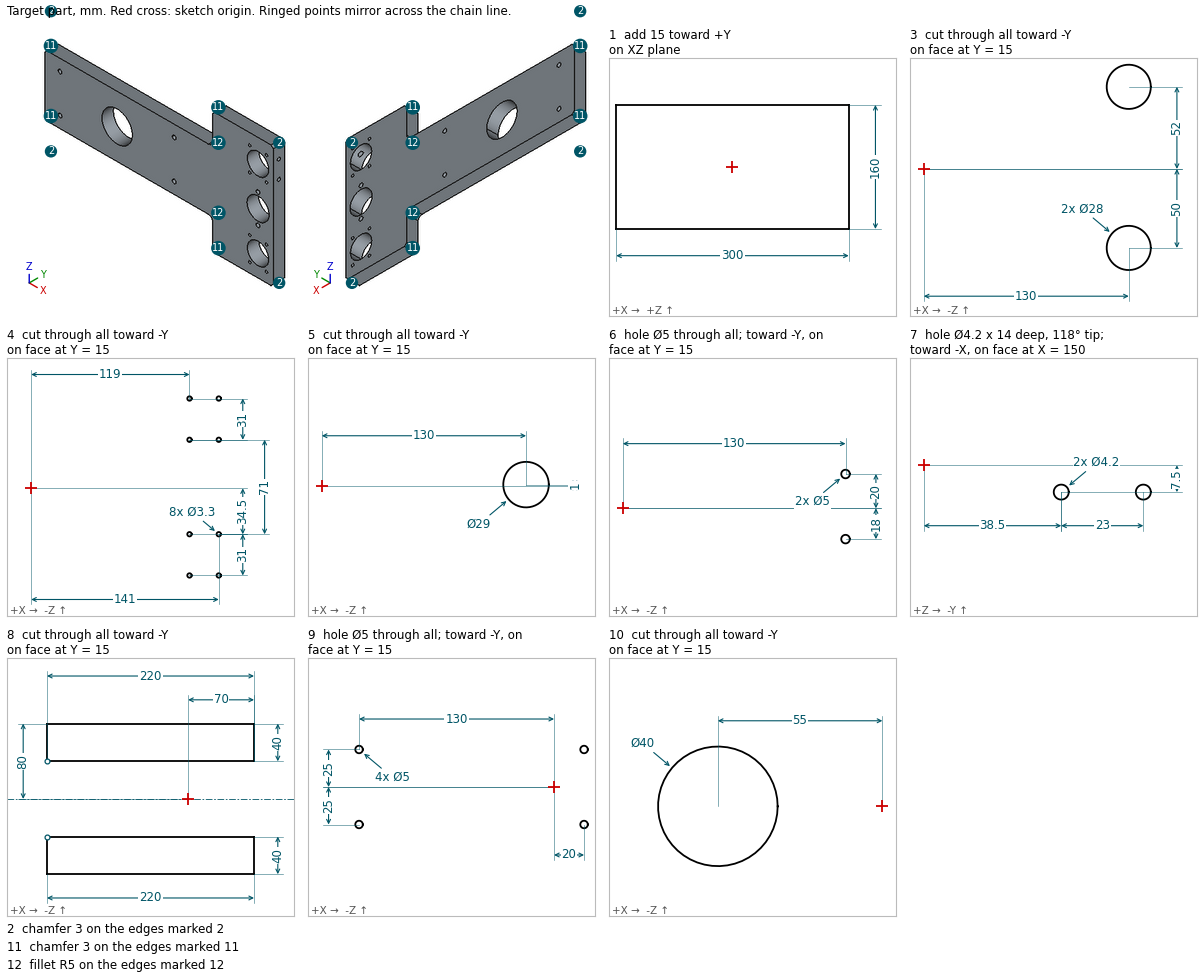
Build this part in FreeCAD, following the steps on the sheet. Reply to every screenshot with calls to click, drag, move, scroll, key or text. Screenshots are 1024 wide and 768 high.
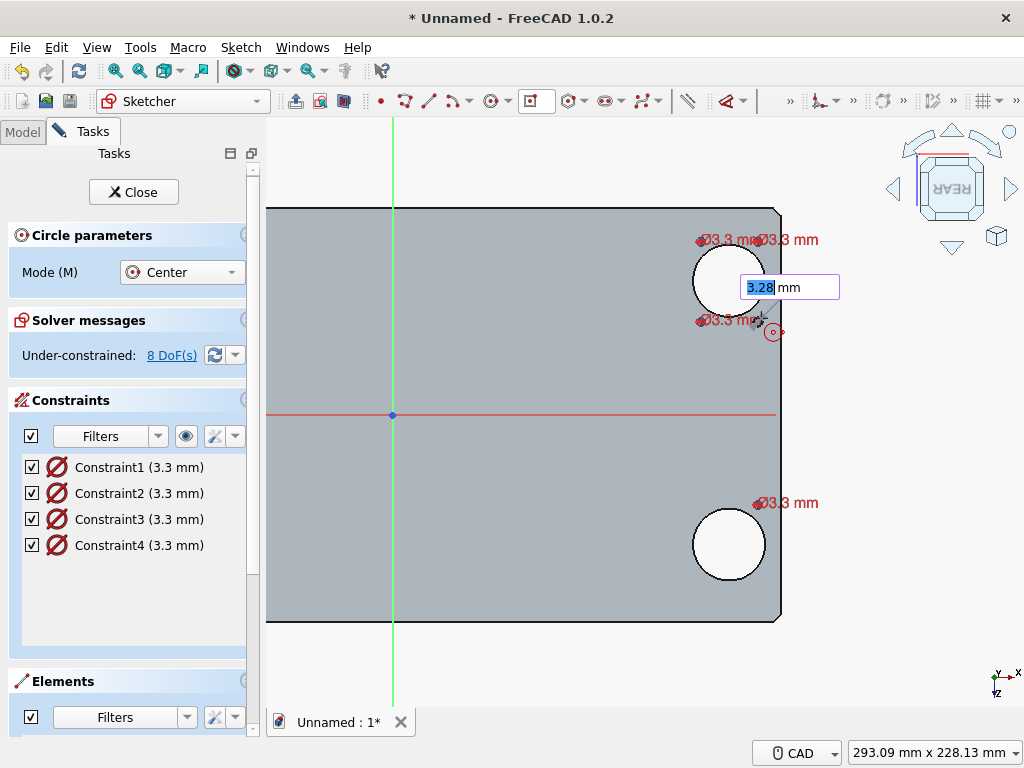
text(3.3)
key(Return)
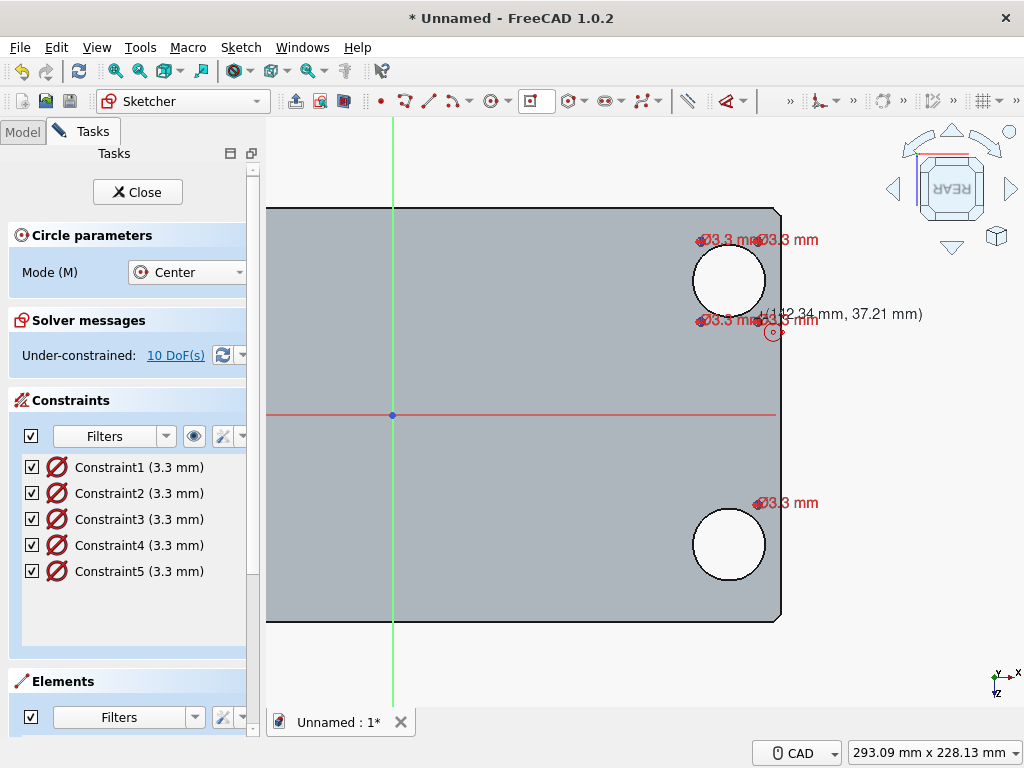
scroll(701, 504, up, 9)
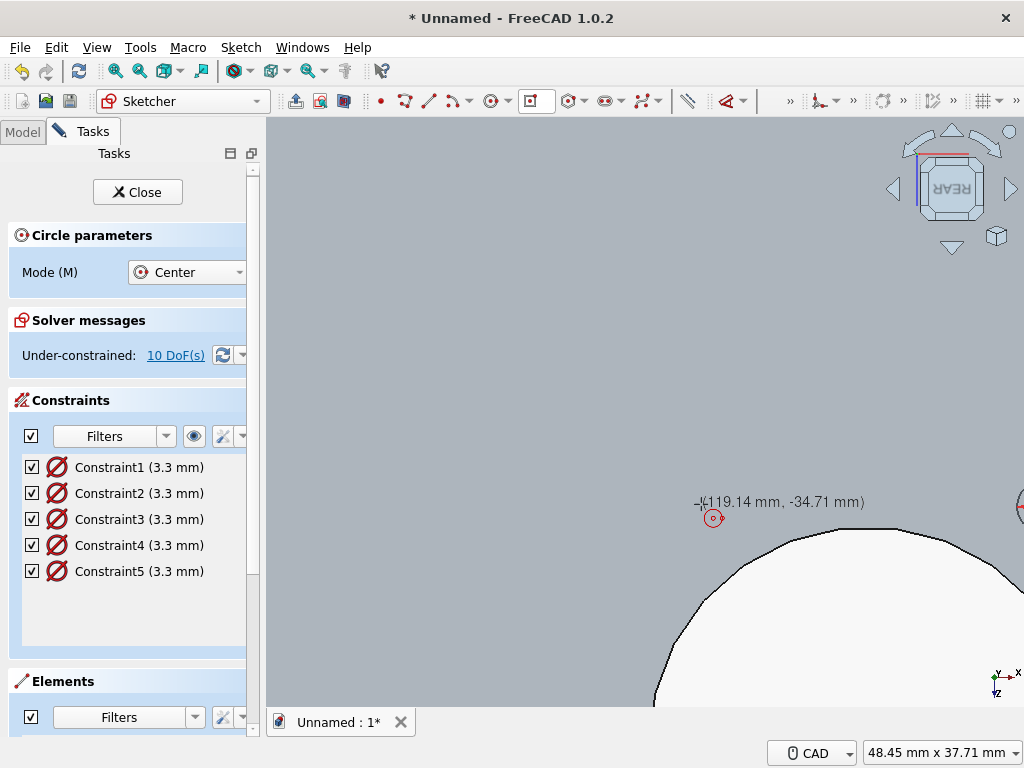
scroll(701, 504, down, 9)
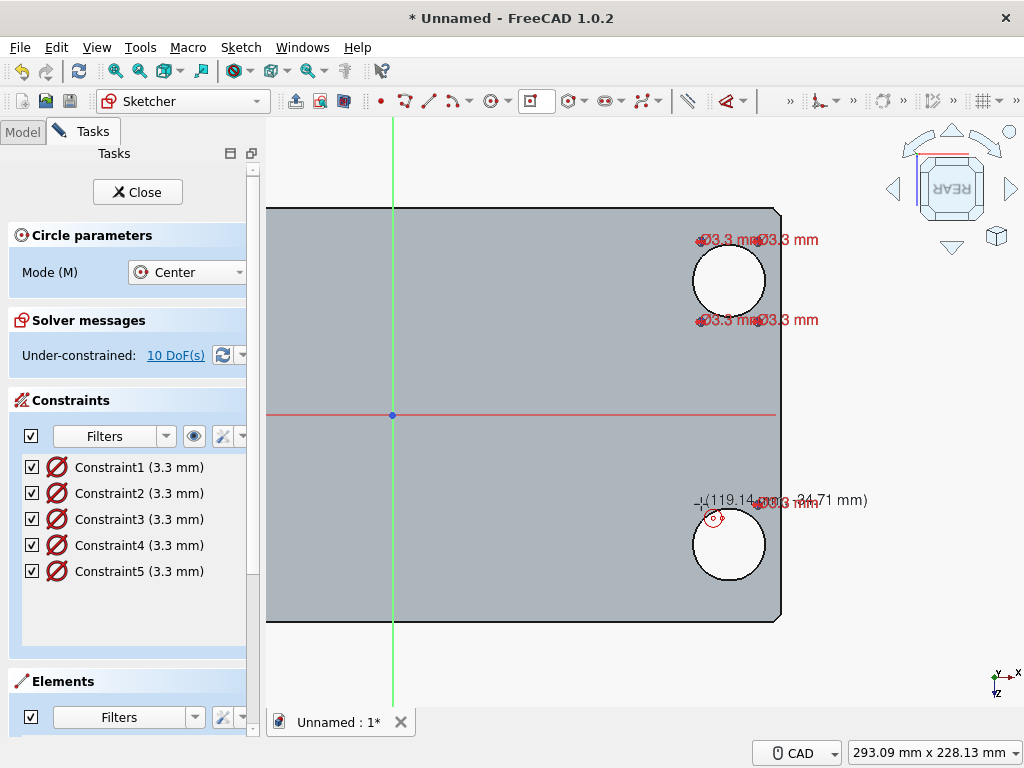
click(701, 504)
move(704, 501)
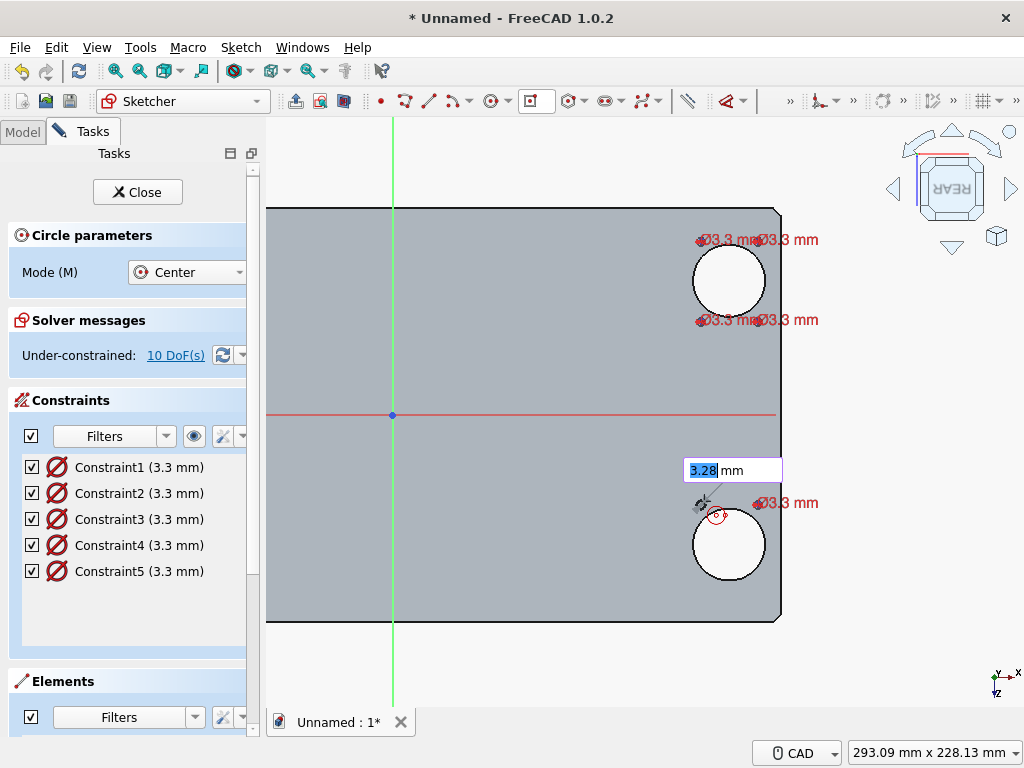
text(3.3)
key(Return)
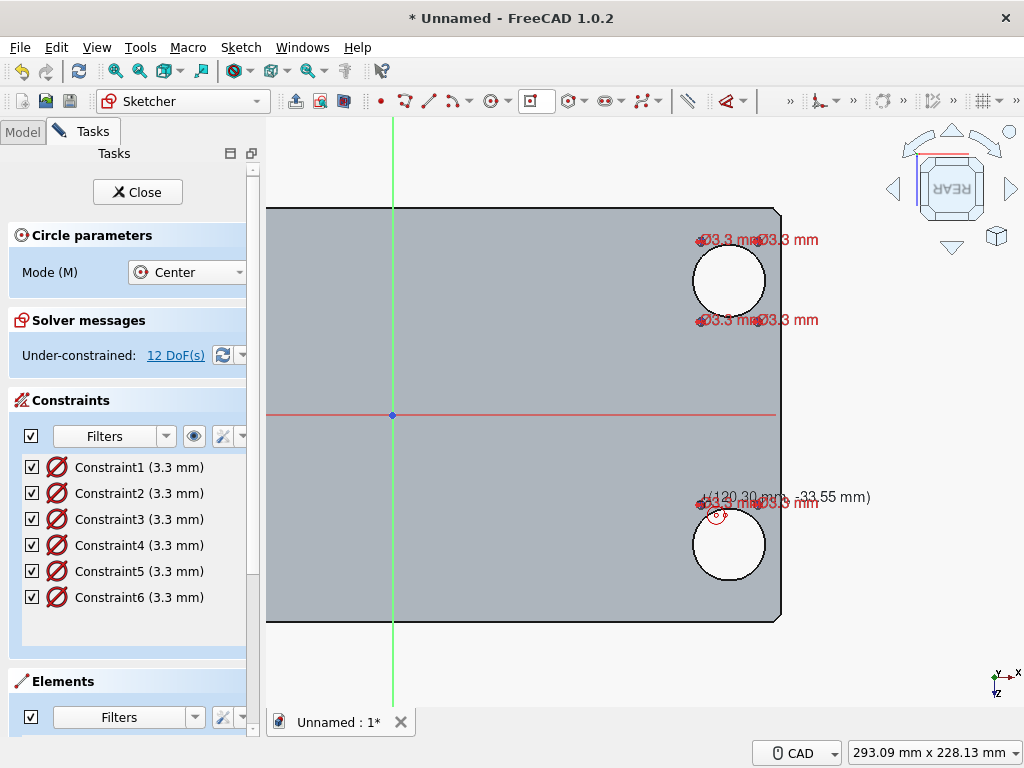
scroll(701, 585, up, 9)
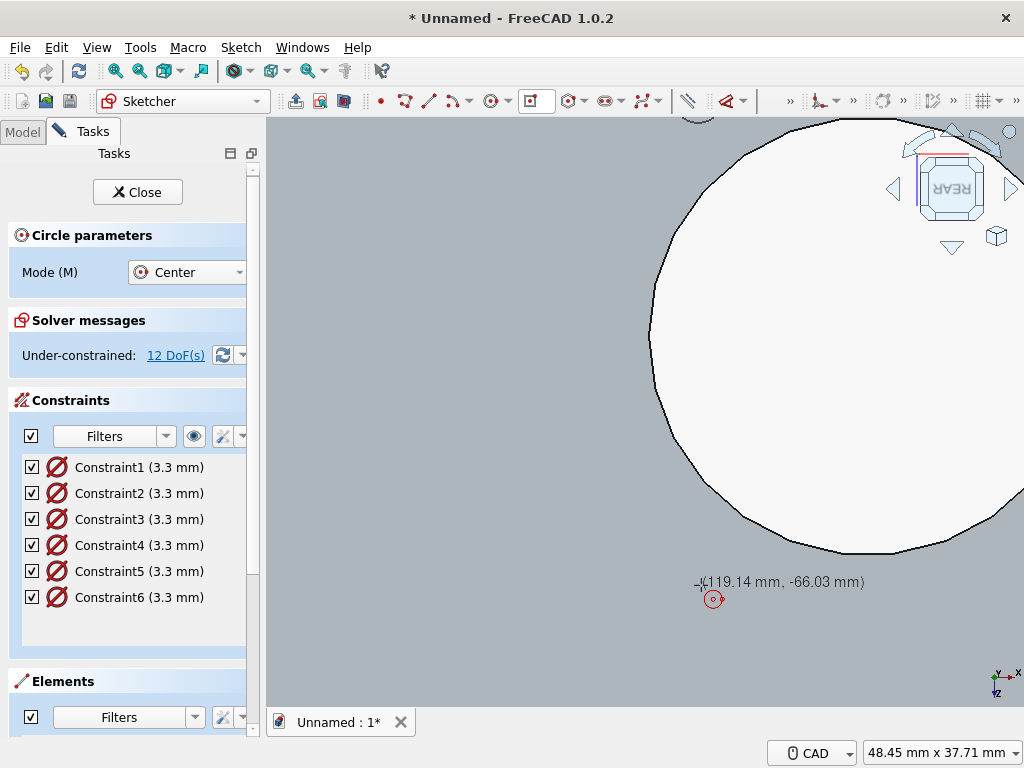
scroll(701, 585, down, 9)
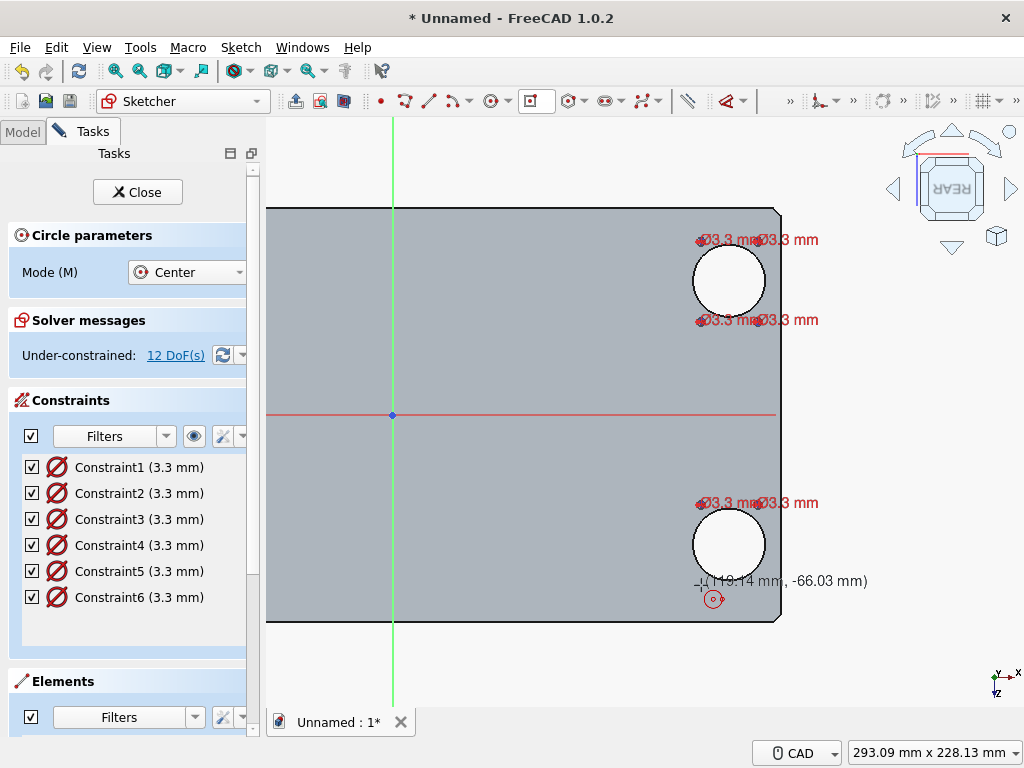
click(701, 585)
move(704, 582)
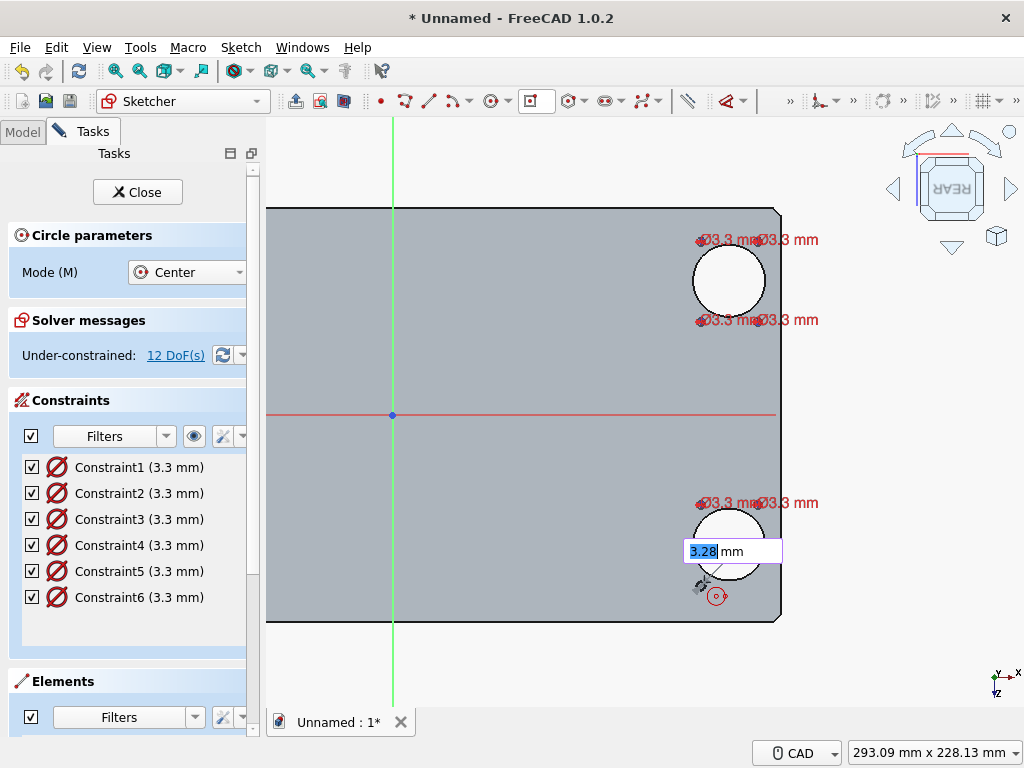
text(3.3)
key(Return)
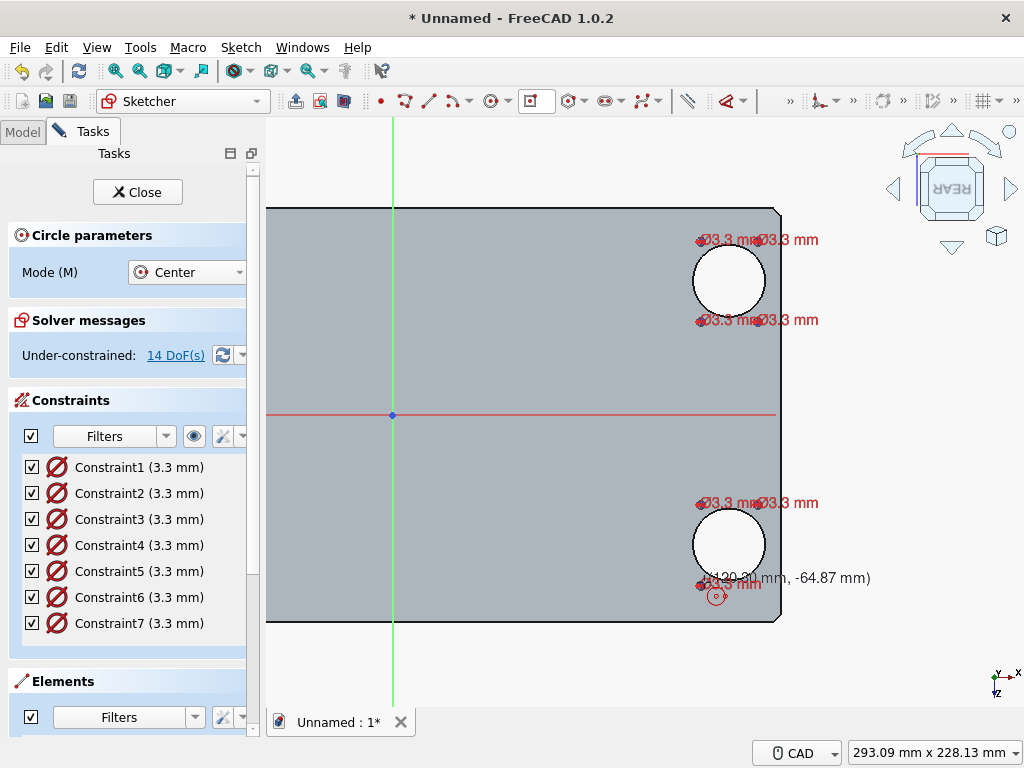
scroll(758, 585, up, 9)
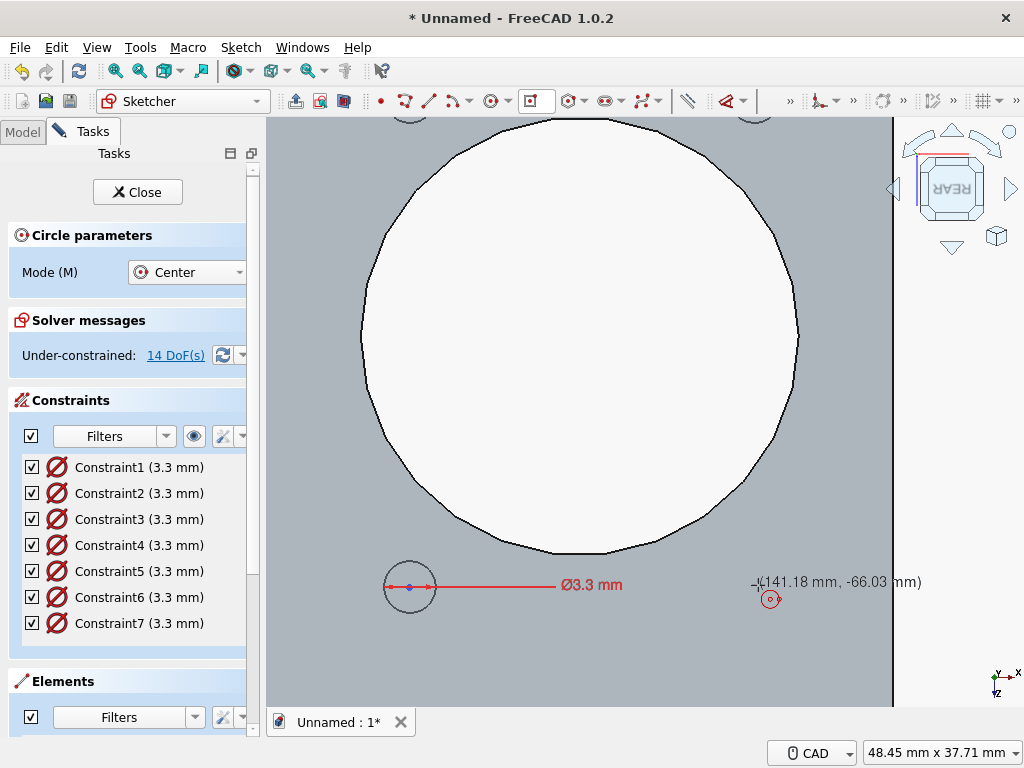
scroll(758, 585, down, 9)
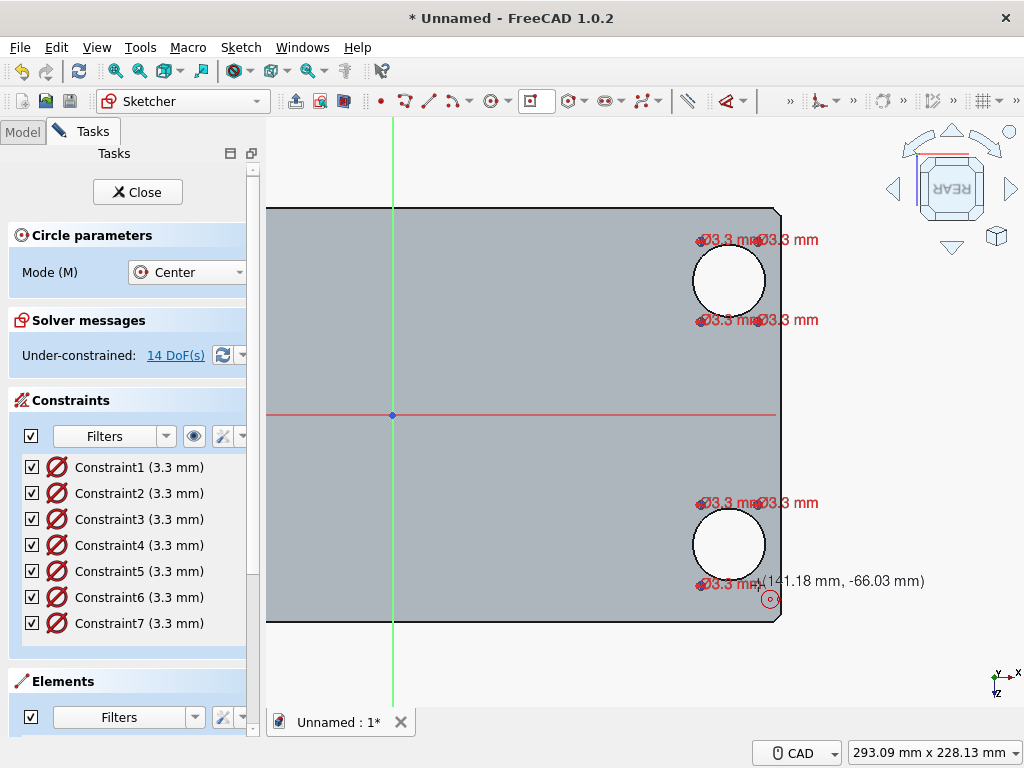
click(758, 585)
move(761, 582)